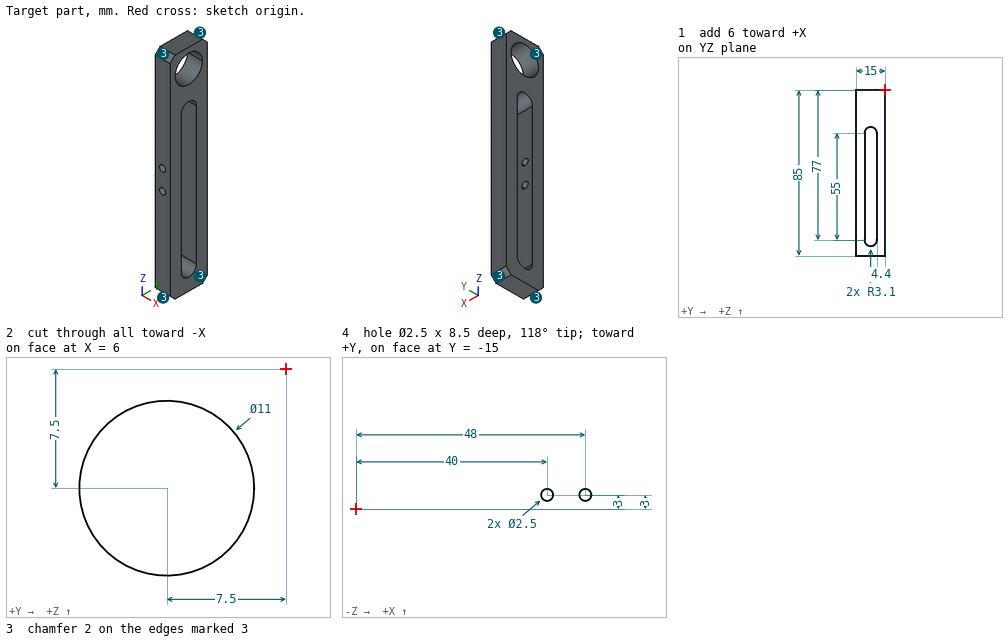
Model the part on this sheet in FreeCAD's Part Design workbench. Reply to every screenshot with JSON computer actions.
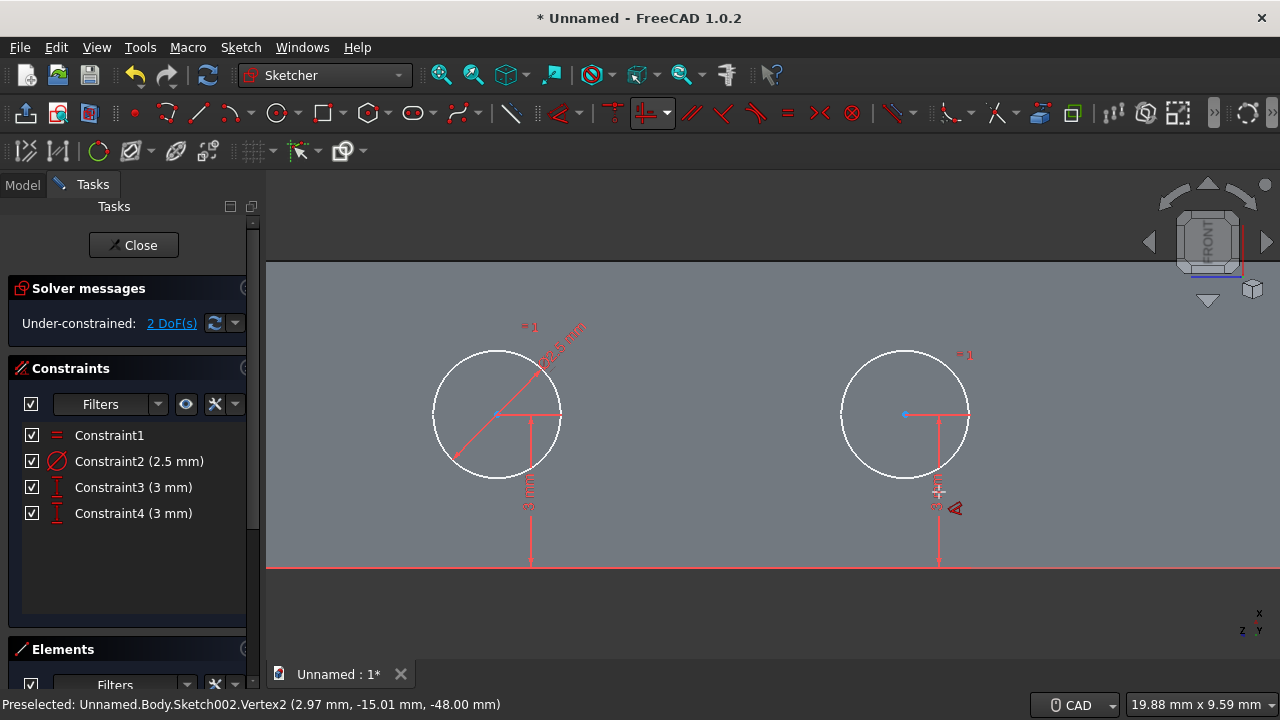
{"action": "left_click", "coordinate": [497, 415]}
{"action": "left_click", "coordinate": [395, 602]}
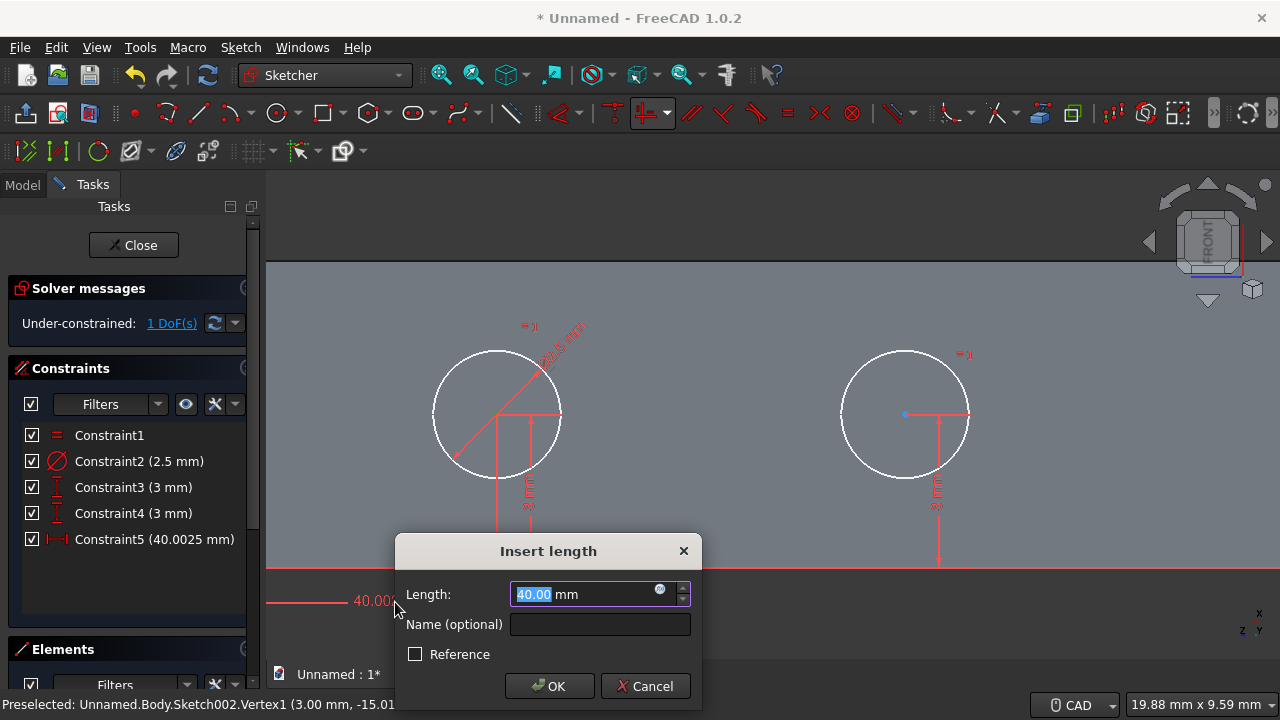
{"action": "type", "text": "40"}
{"action": "key", "text": "Return"}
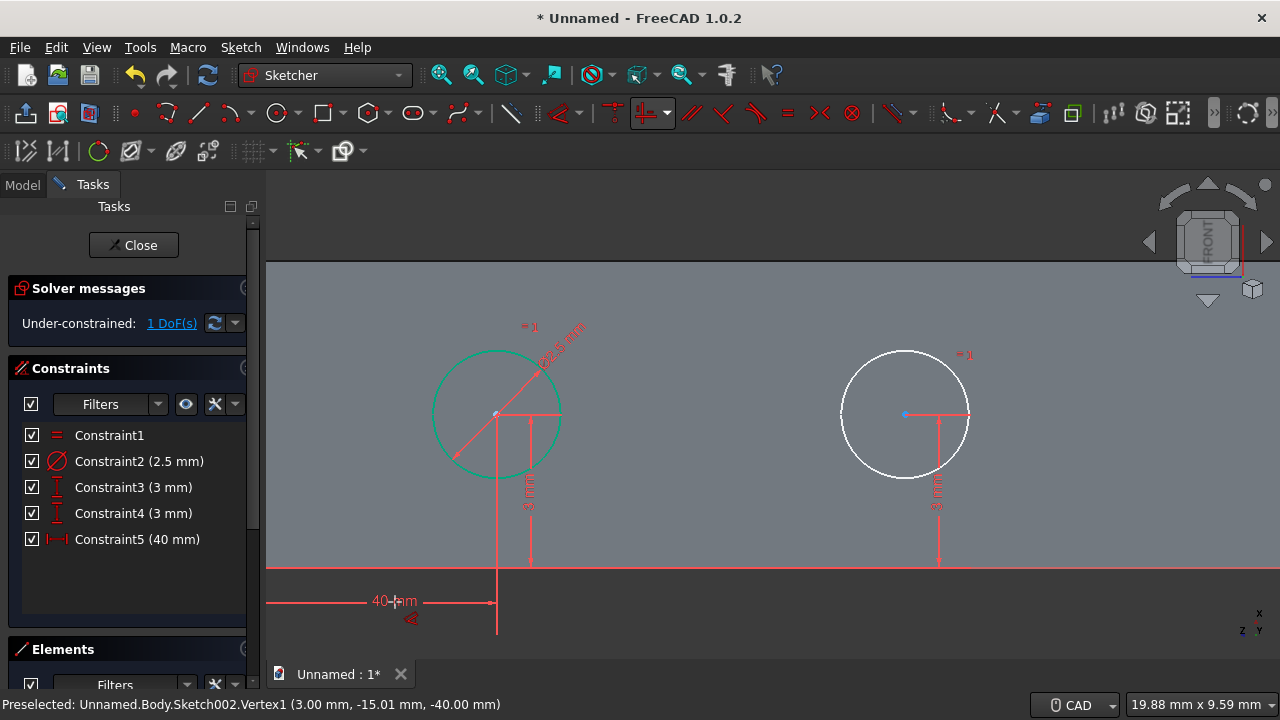
{"action": "left_click", "coordinate": [905, 415]}
{"action": "left_click", "coordinate": [599, 602]}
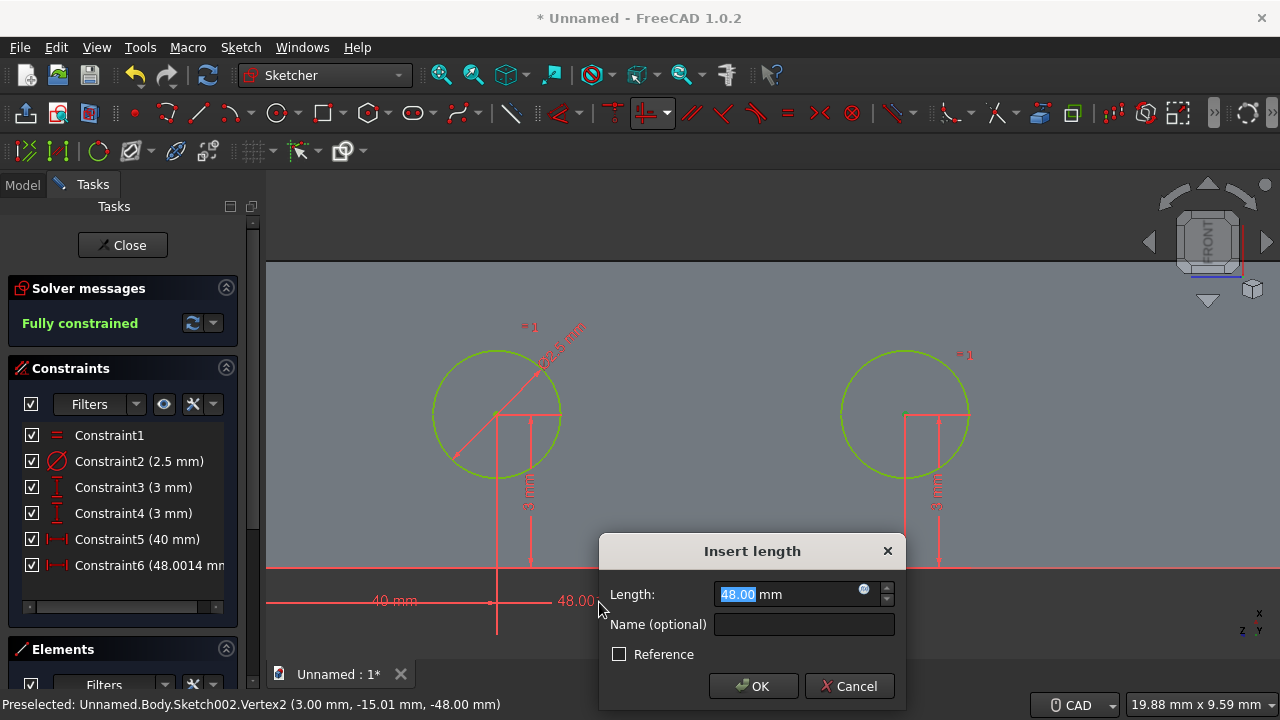
{"action": "type", "text": "48"}
{"action": "key", "text": "Return"}
{"action": "key", "text": "Escape"}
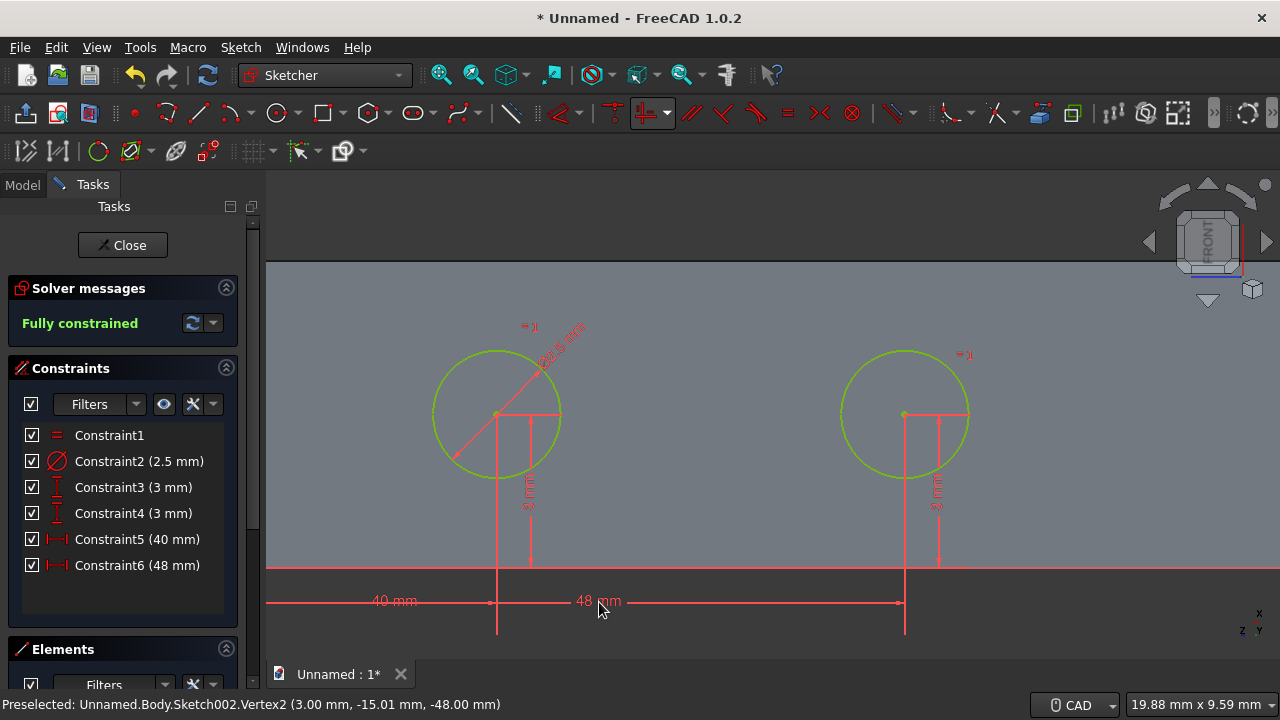
{"action": "left_click", "coordinate": [123, 245]}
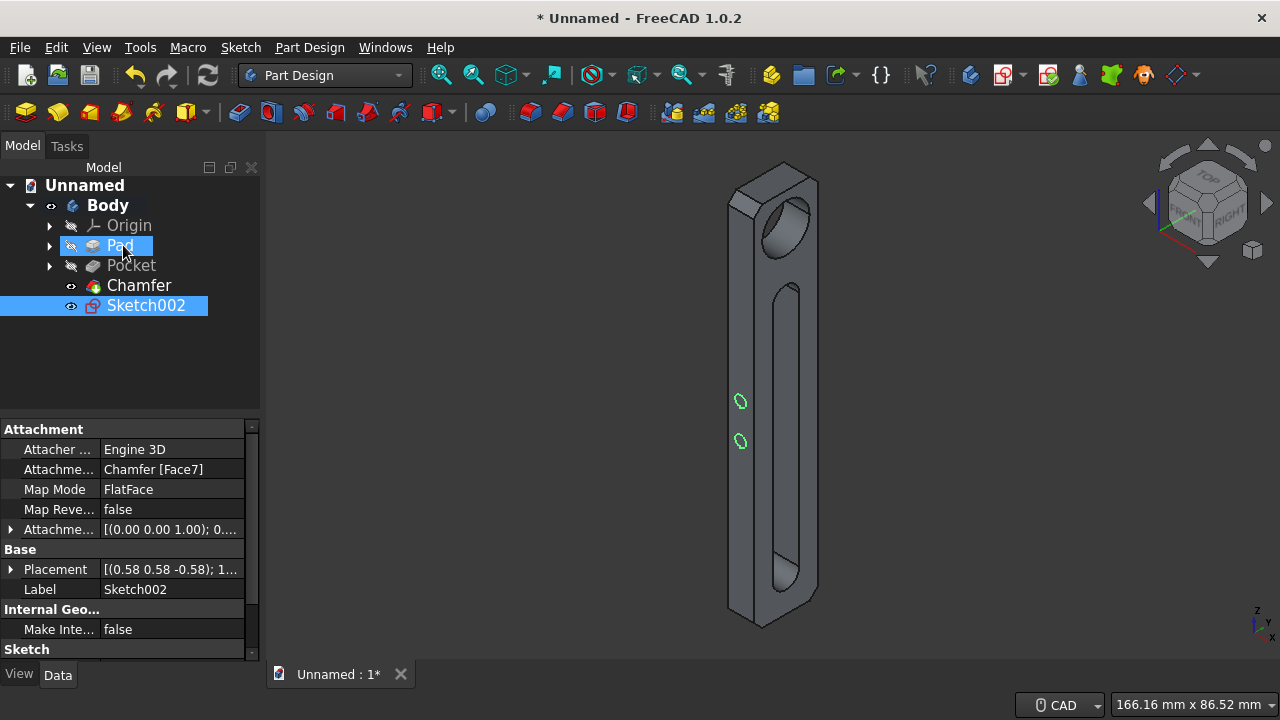
{"action": "left_click", "coordinate": [272, 112]}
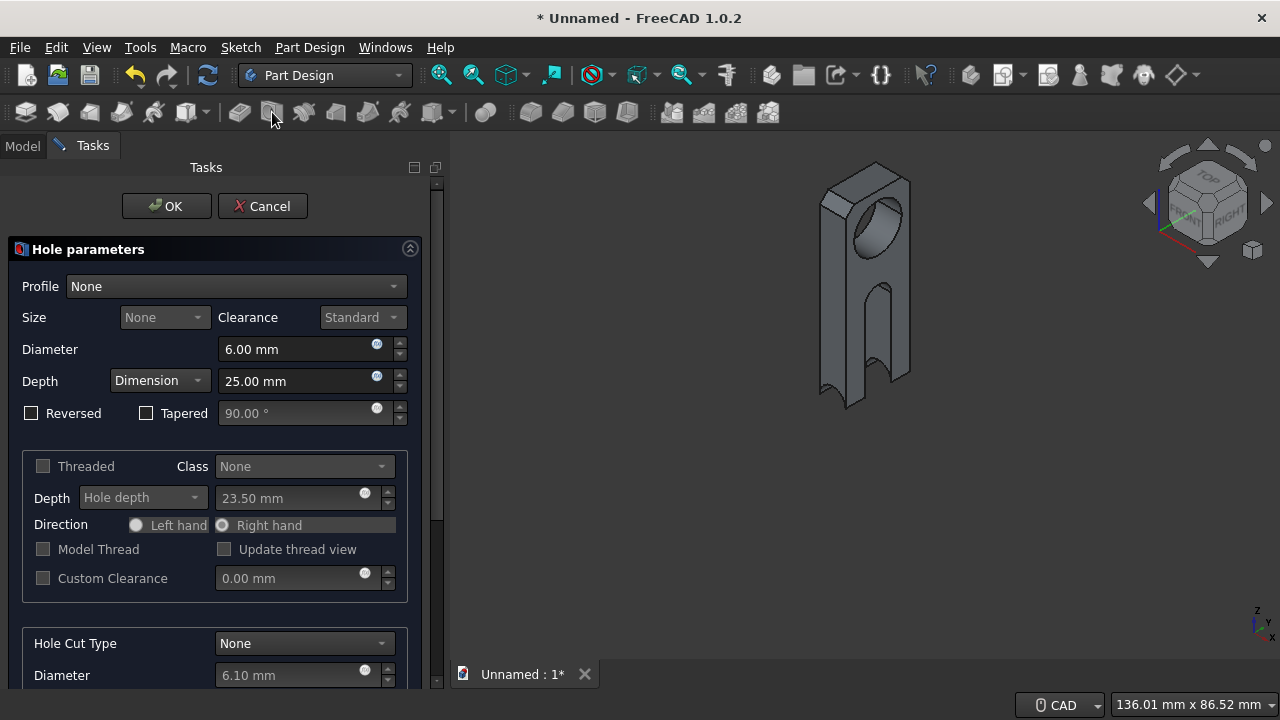
{"action": "triple_click", "coordinate": [305, 349]}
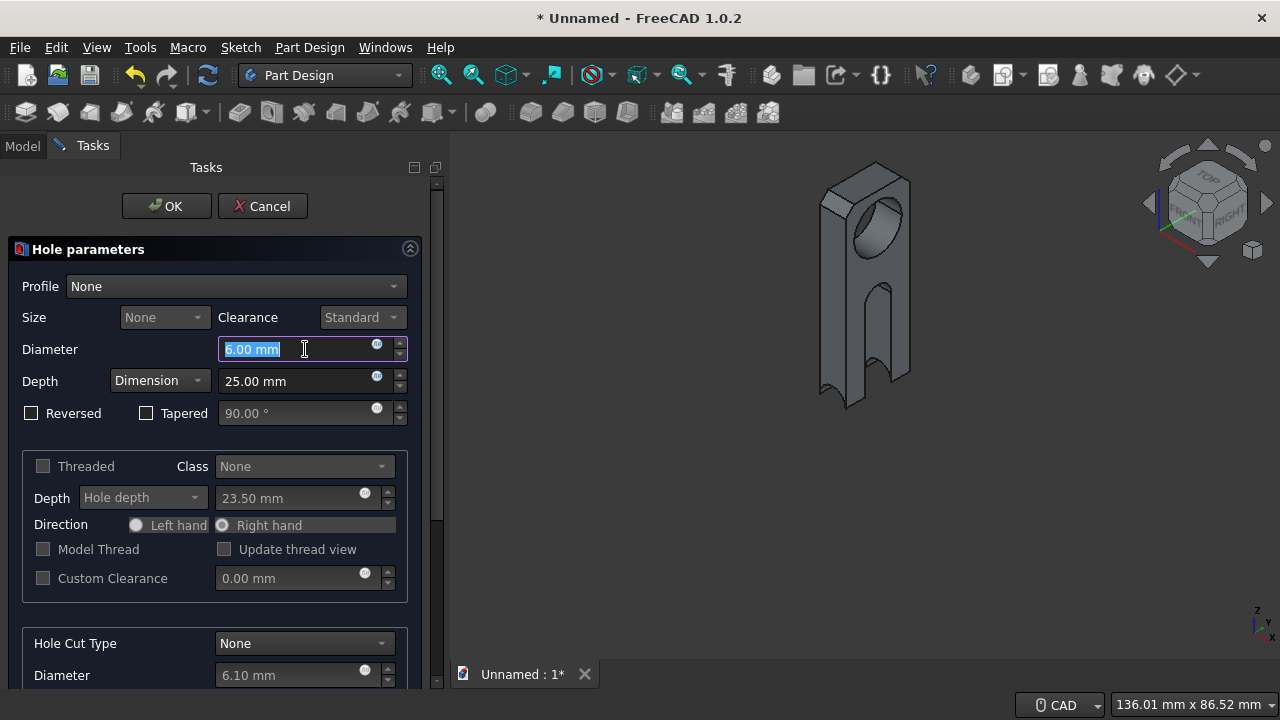
{"action": "type", "text": "2.5"}
{"action": "key", "text": "Tab"}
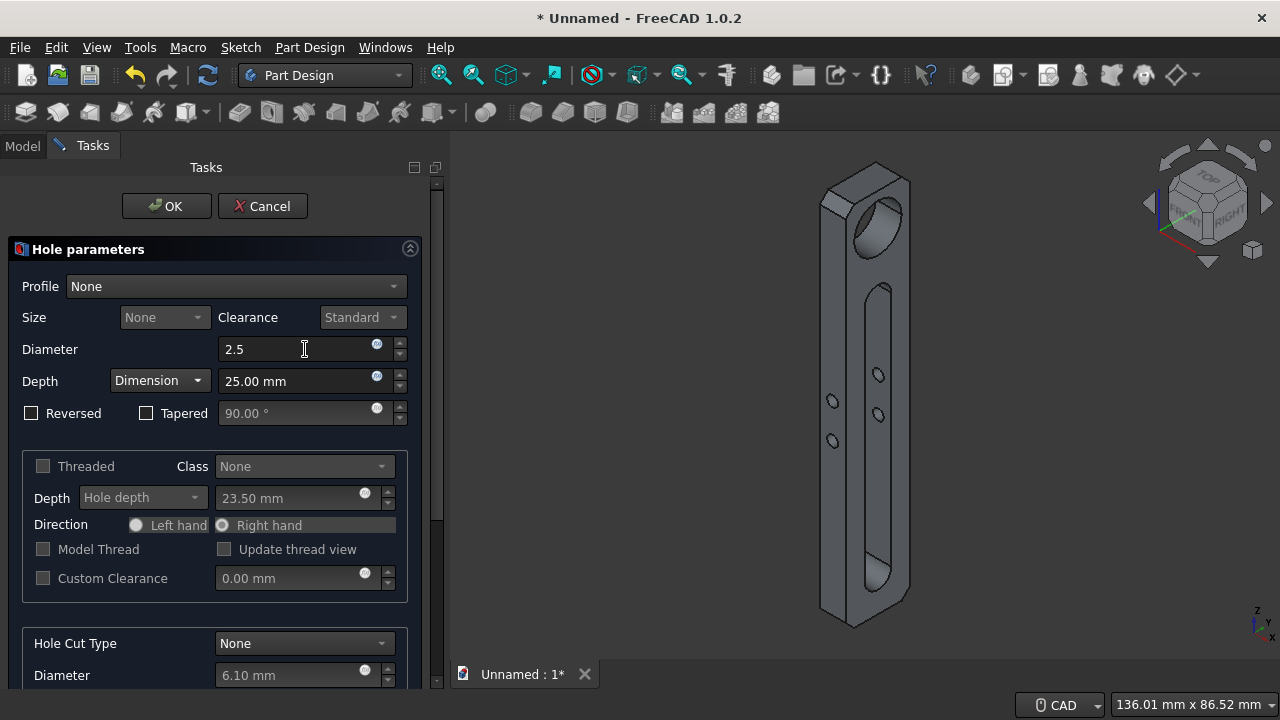
{"action": "triple_click", "coordinate": [305, 381]}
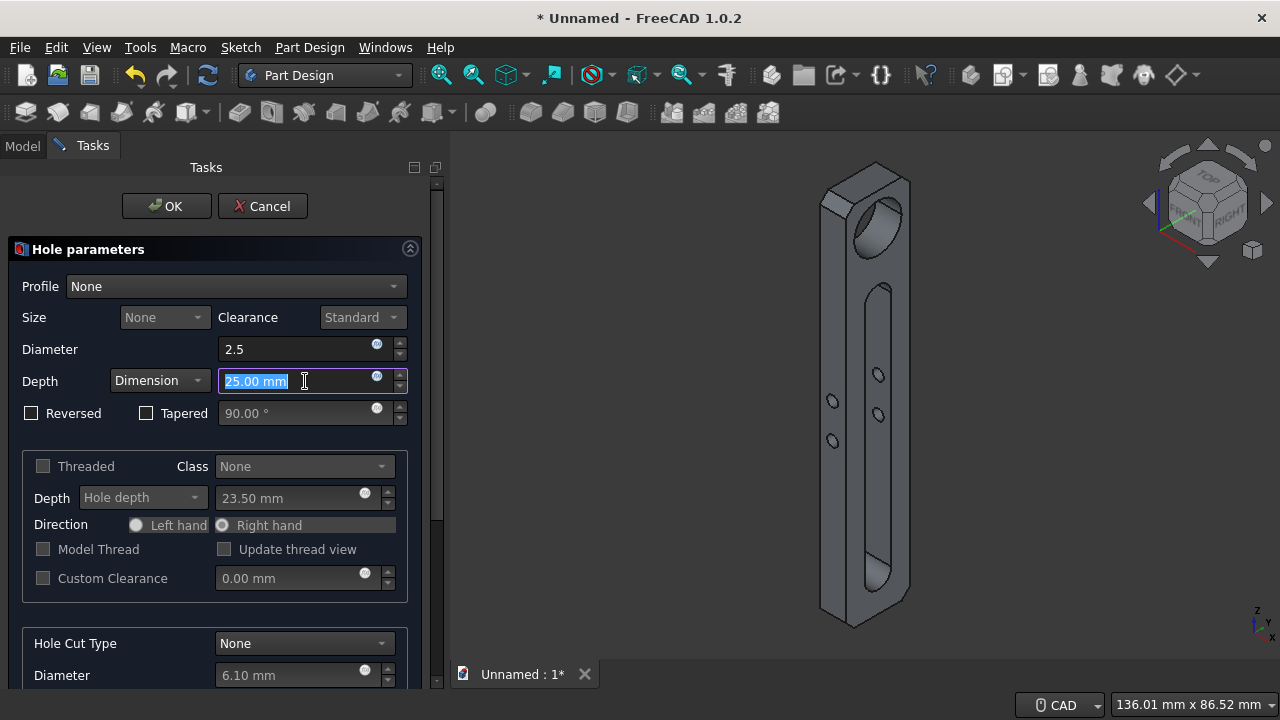
{"action": "type", "text": "8.5"}
{"action": "key", "text": "Tab"}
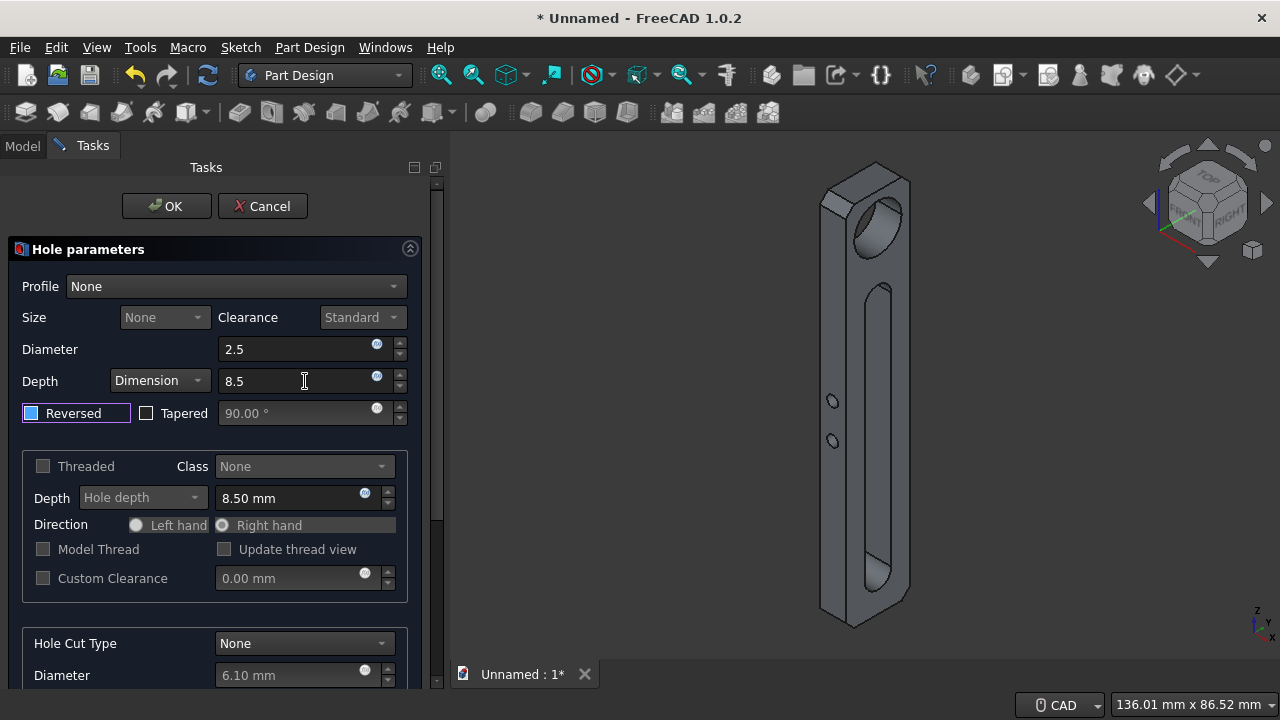
{"action": "left_click", "coordinate": [167, 206]}